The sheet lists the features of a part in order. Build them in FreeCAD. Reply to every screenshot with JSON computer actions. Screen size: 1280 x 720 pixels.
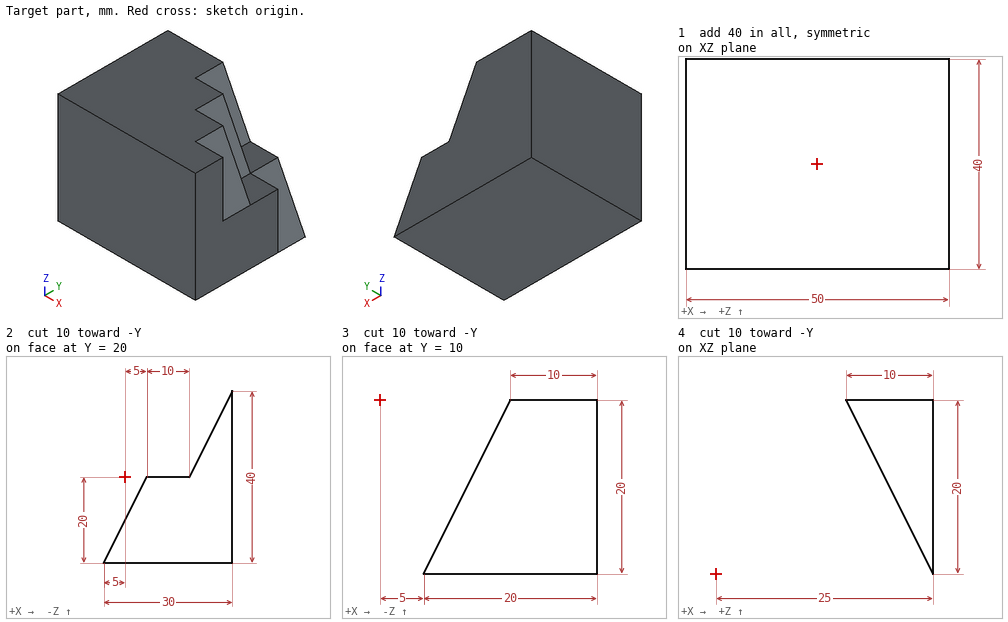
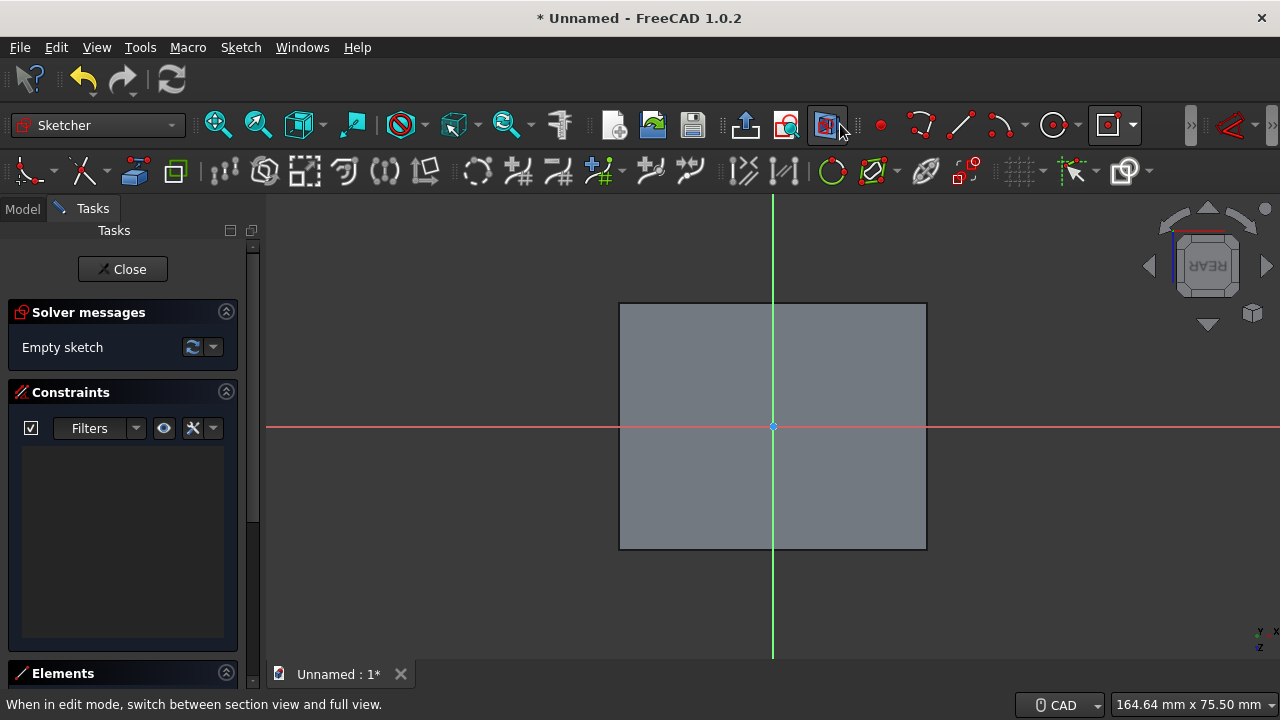
{"action": "left_click", "coordinate": [922, 126]}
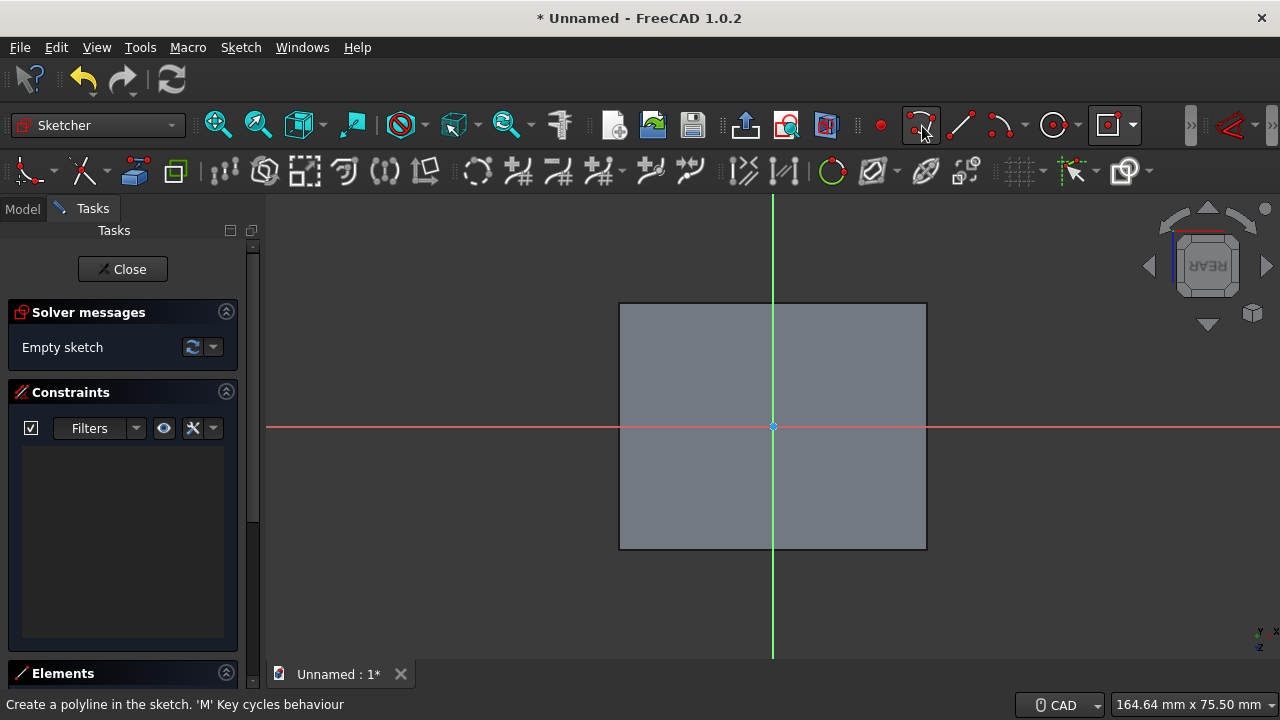
{"action": "left_click", "coordinate": [804, 426]}
{"action": "left_click", "coordinate": [742, 550]}
{"action": "left_click", "coordinate": [927, 550]}
{"action": "left_click", "coordinate": [927, 303]}
{"action": "left_click", "coordinate": [865, 418]}
{"action": "left_click", "coordinate": [804, 426]}
{"action": "key", "text": "Escape"}
{"action": "key", "text": "Escape"}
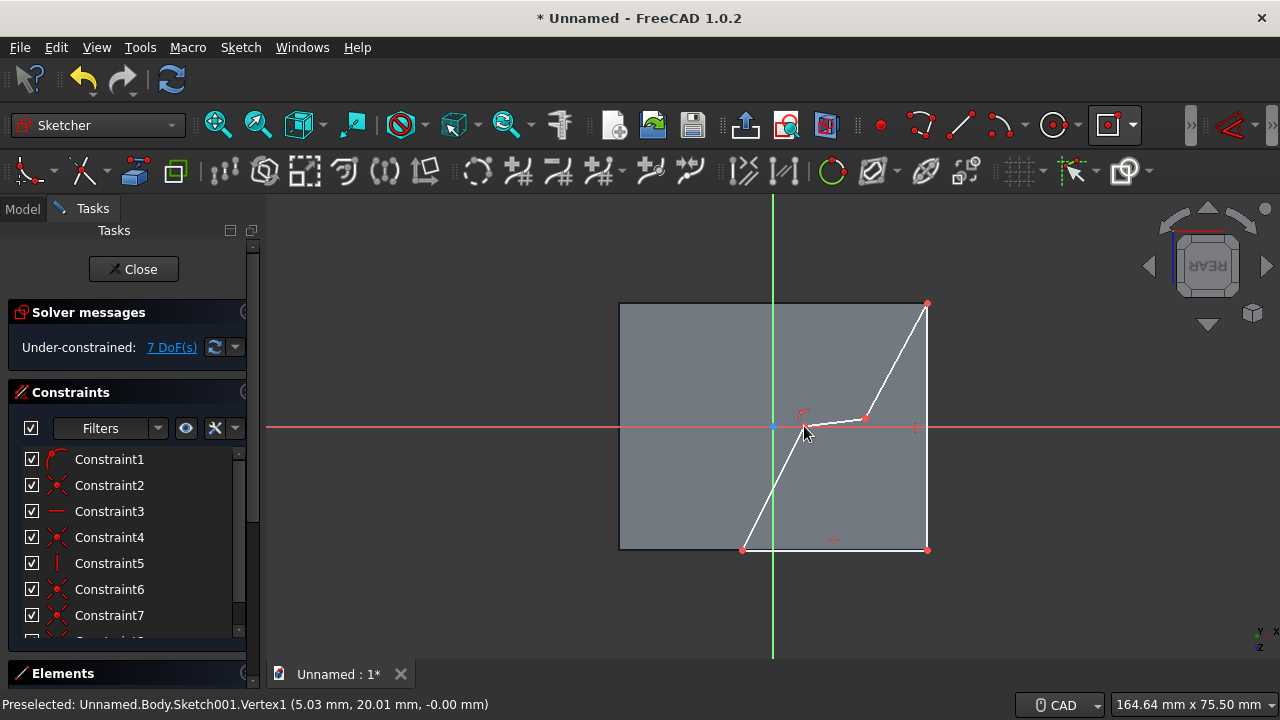
{"action": "left_click", "coordinate": [822, 424]}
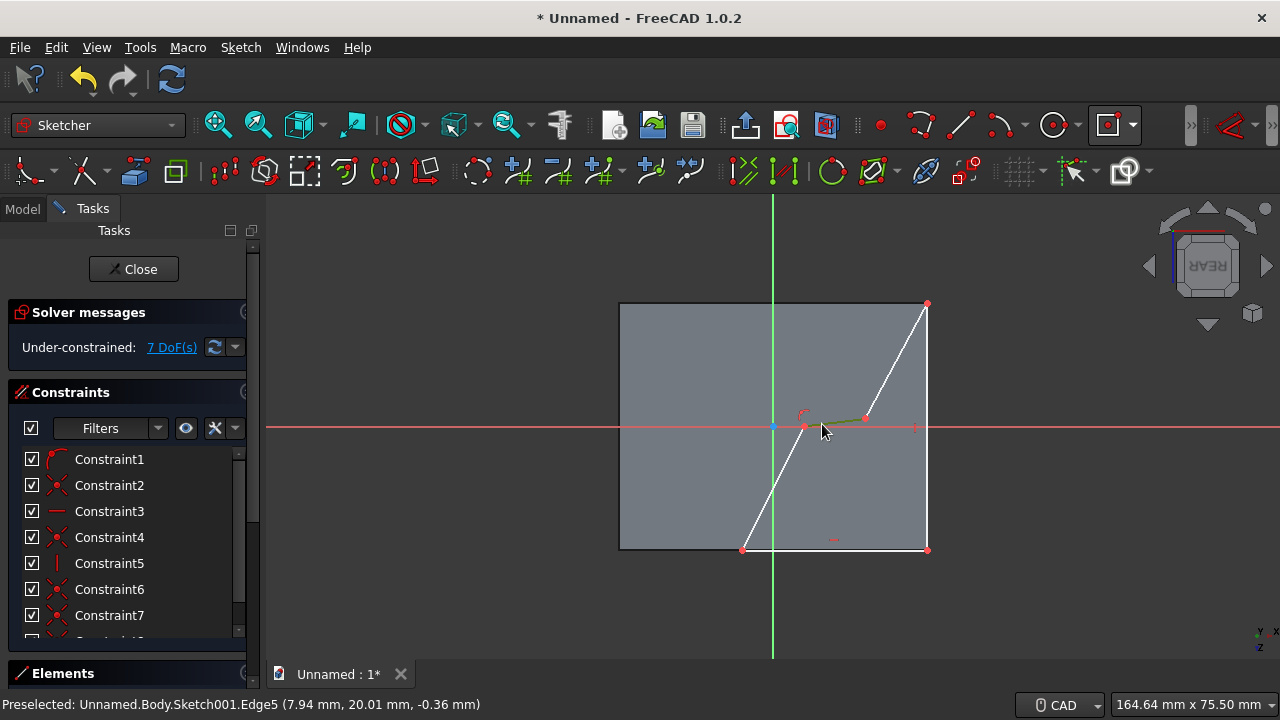
{"action": "key", "text": "h"}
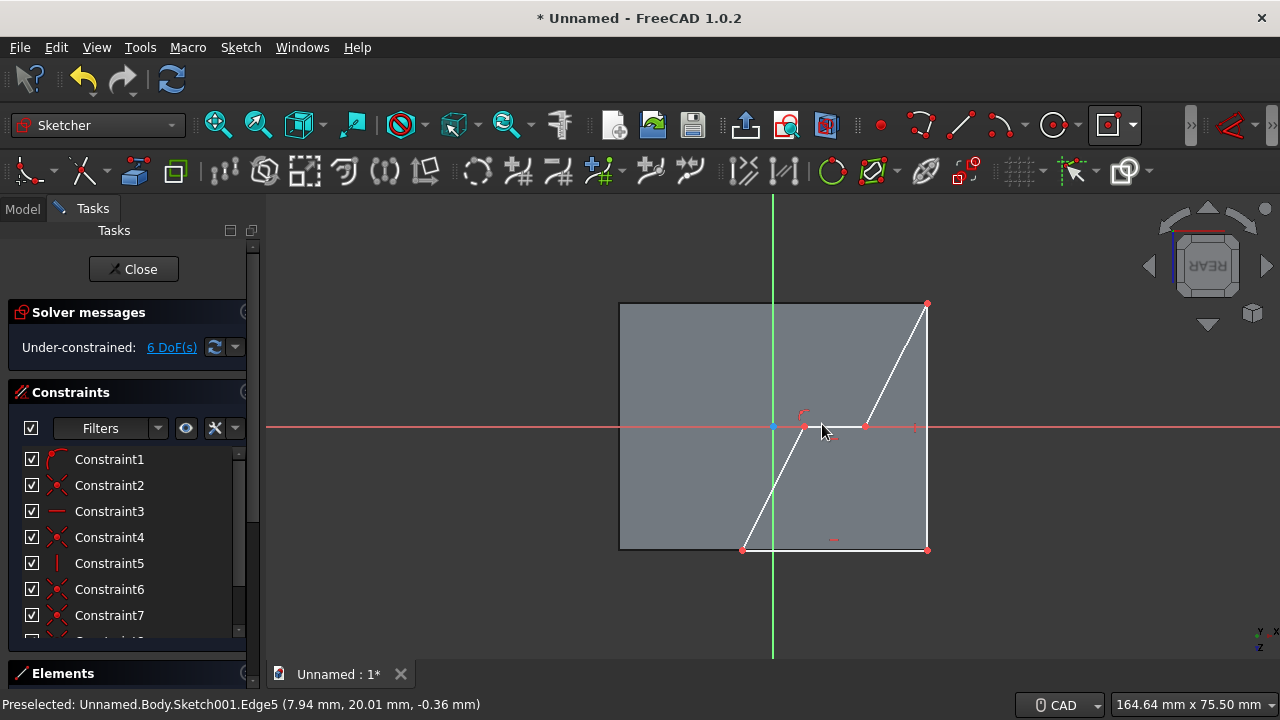
{"action": "left_click", "coordinate": [1230, 126]}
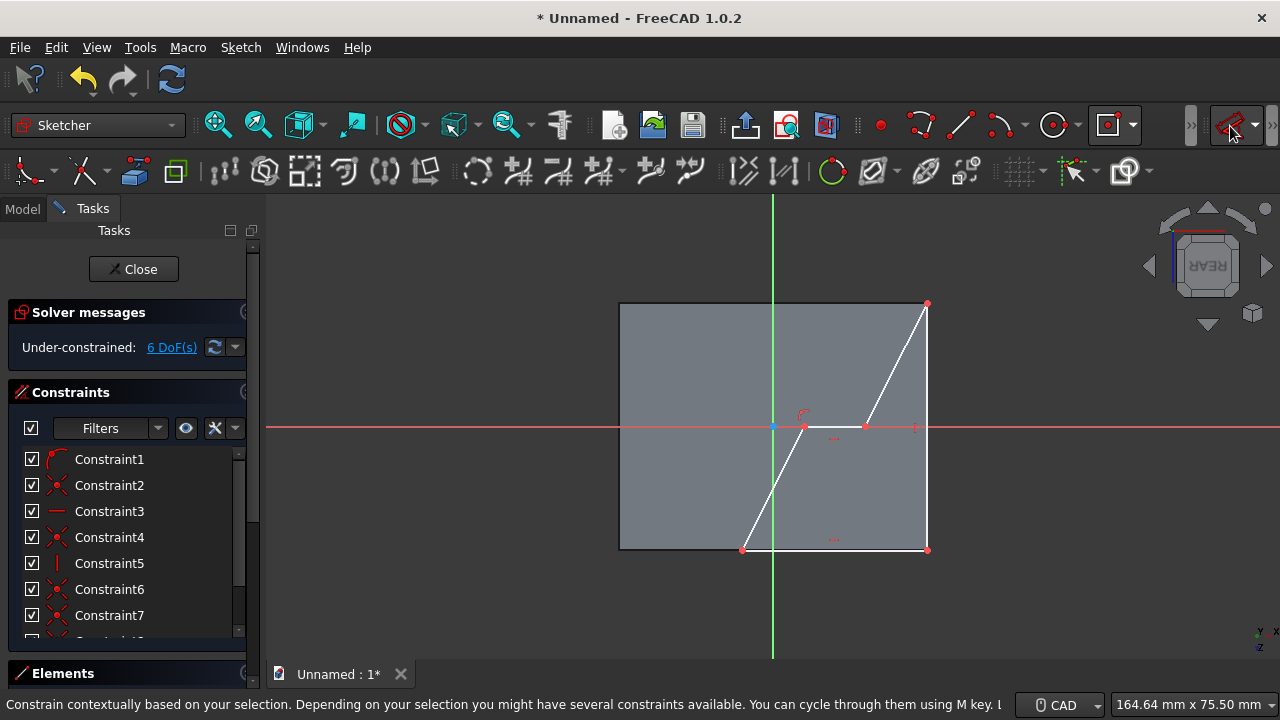
{"action": "left_click", "coordinate": [798, 551]}
{"action": "left_click", "coordinate": [835, 585]}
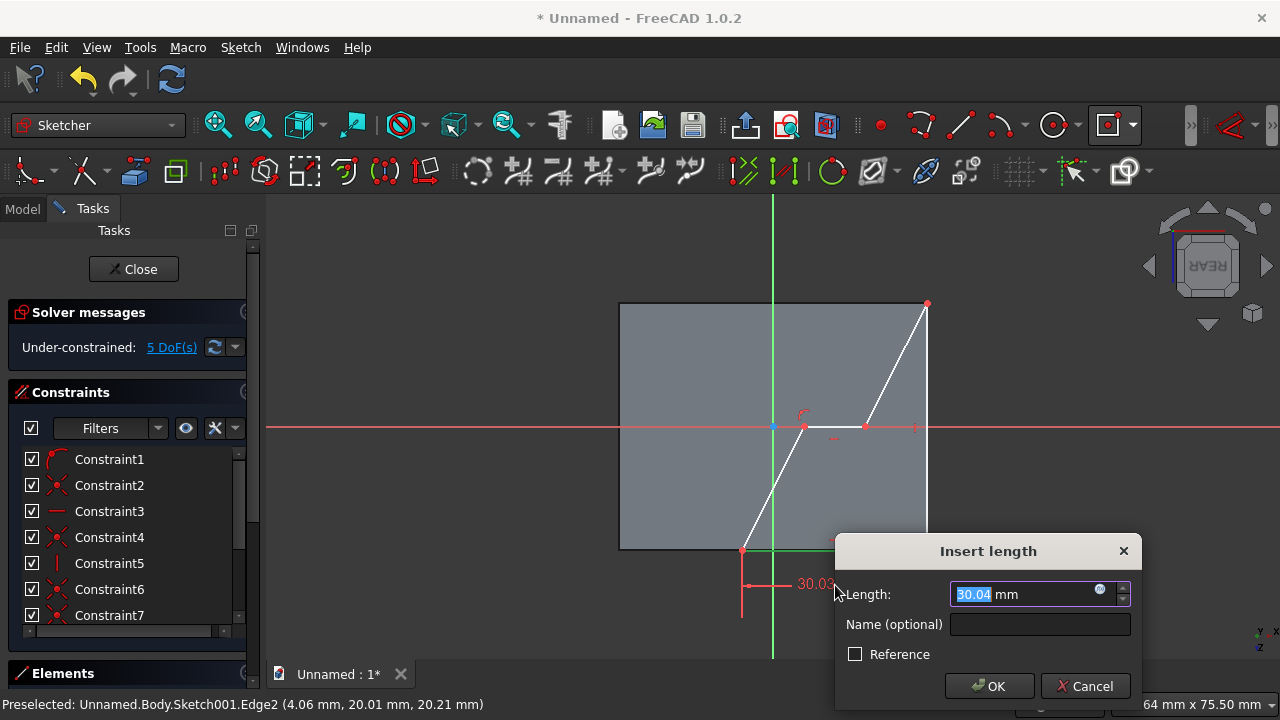
{"action": "type", "text": "30"}
{"action": "key", "text": "Return"}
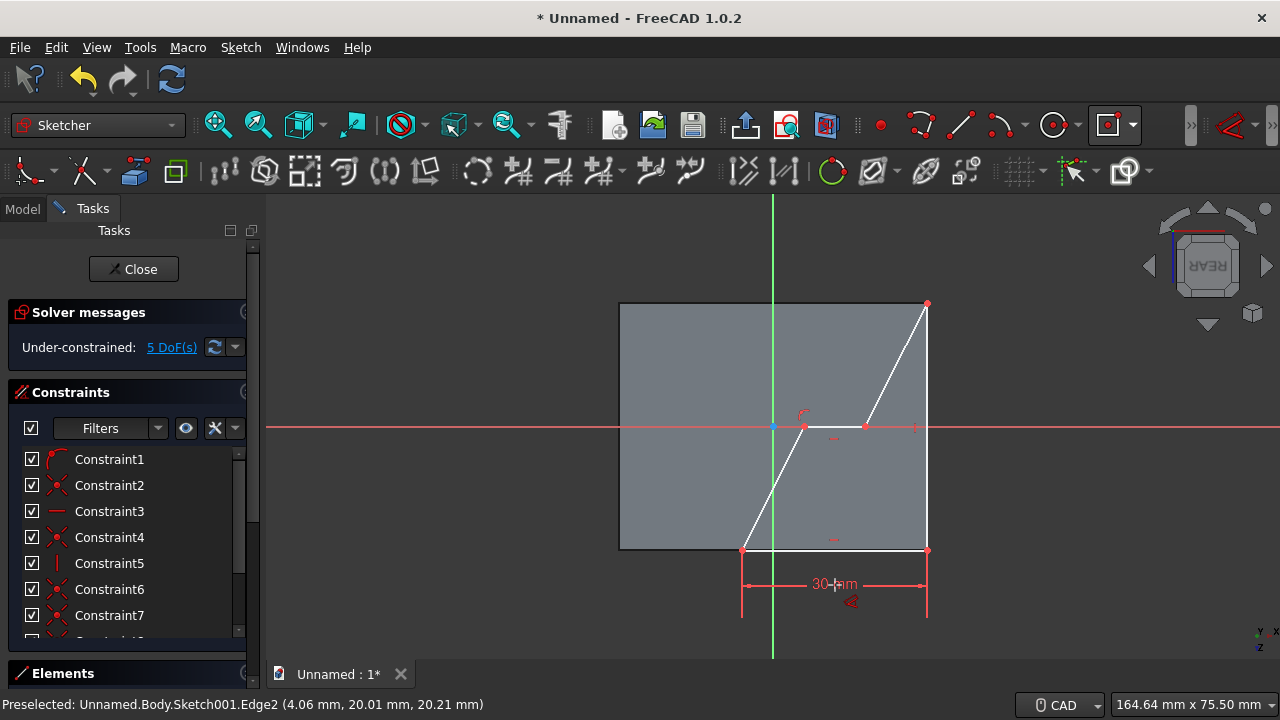
{"action": "left_click", "coordinate": [927, 477]}
{"action": "left_click", "coordinate": [961, 371]}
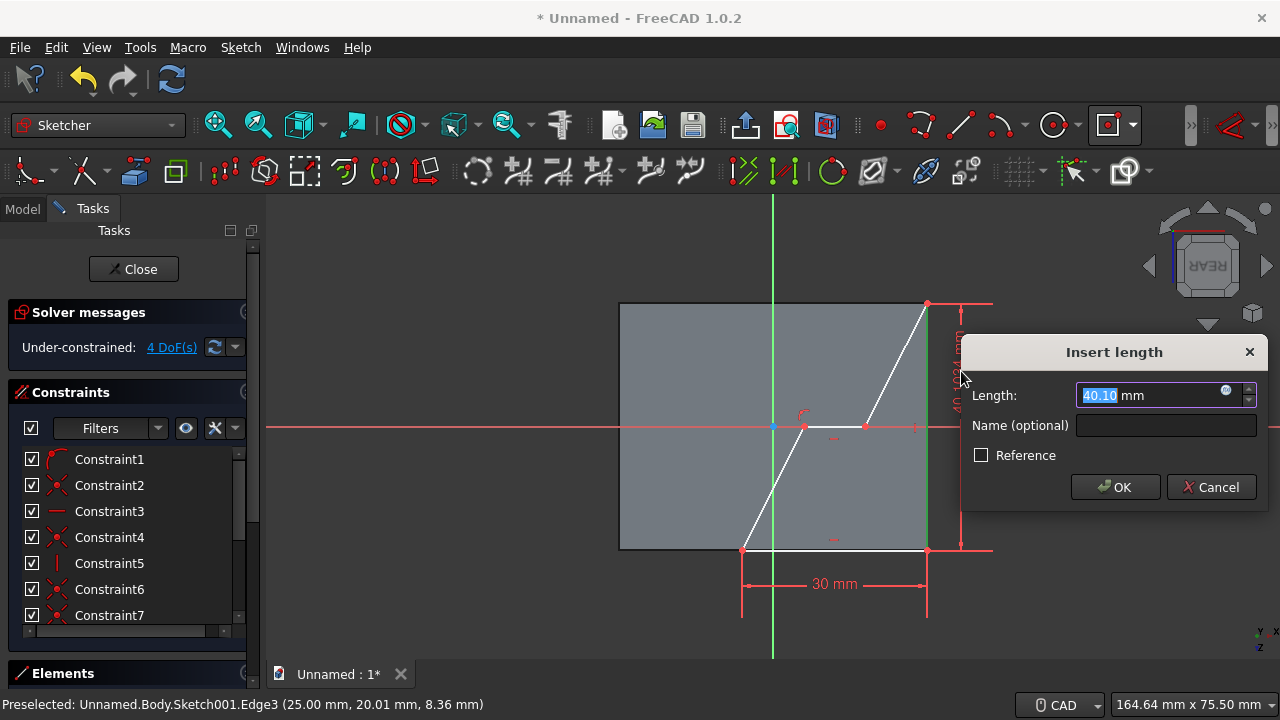
{"action": "type", "text": "40"}
{"action": "key", "text": "Return"}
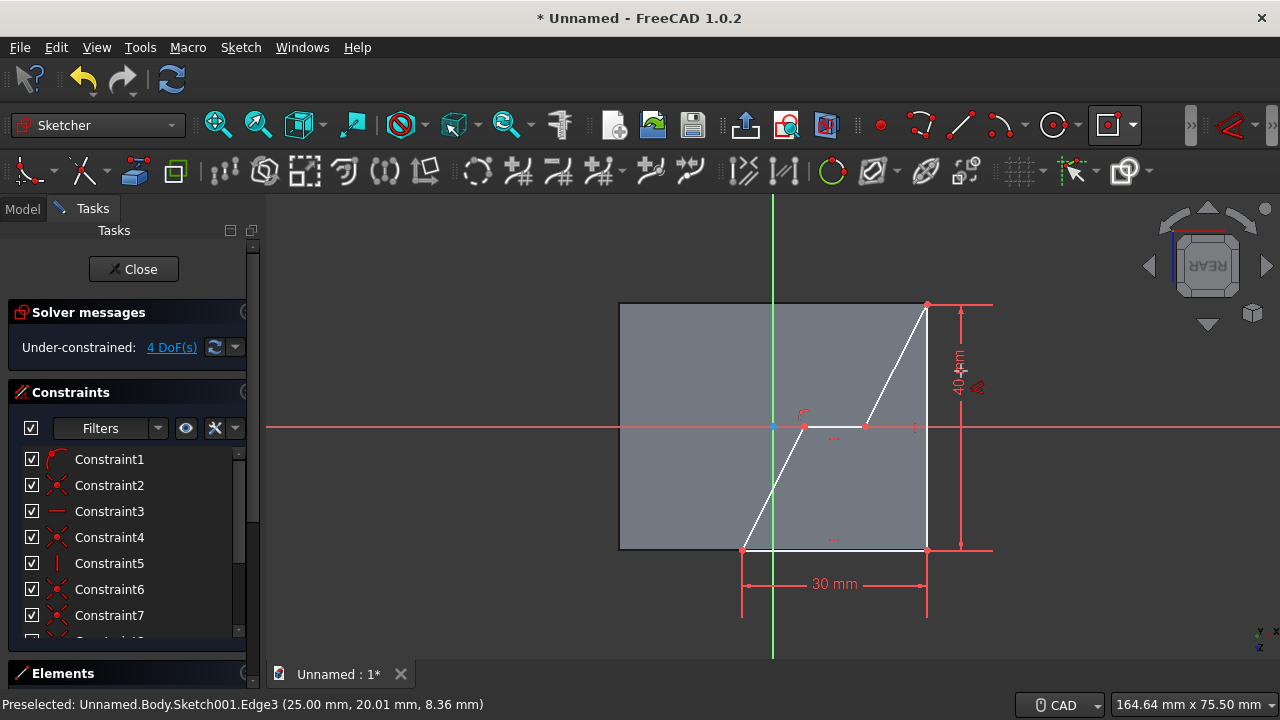
{"action": "left_click", "coordinate": [847, 426]}
{"action": "left_click", "coordinate": [834, 460]}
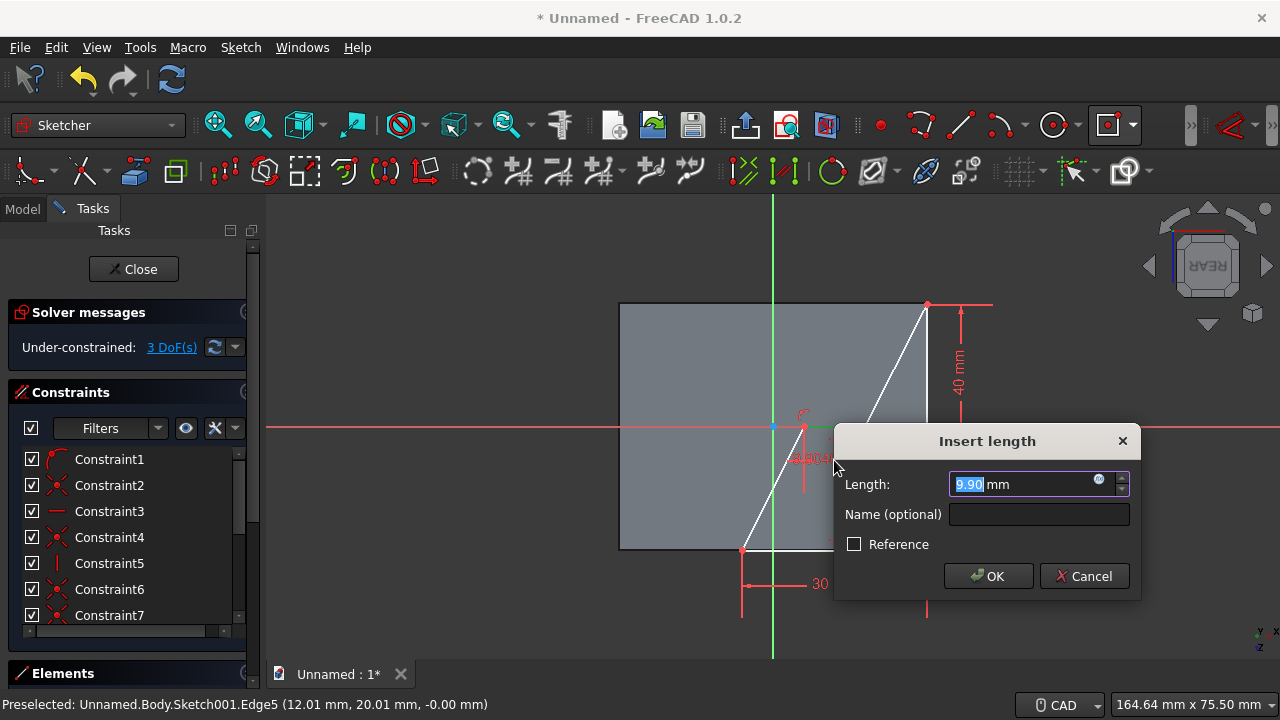
{"action": "type", "text": "10"}
{"action": "key", "text": "Return"}